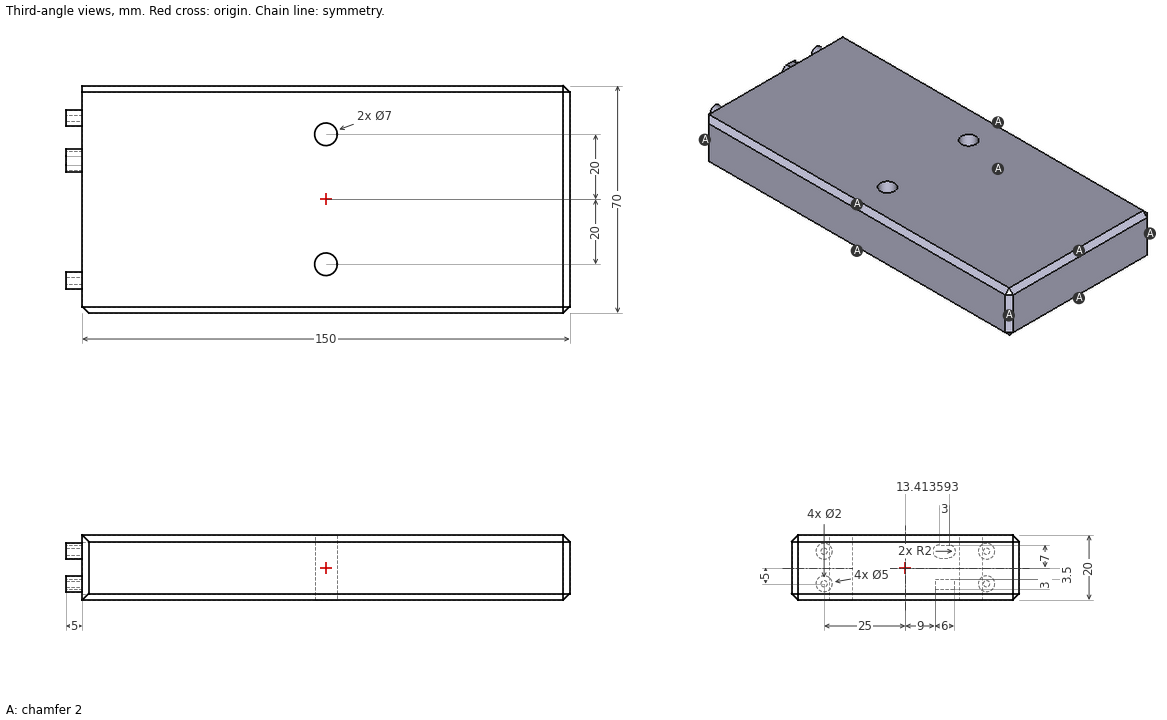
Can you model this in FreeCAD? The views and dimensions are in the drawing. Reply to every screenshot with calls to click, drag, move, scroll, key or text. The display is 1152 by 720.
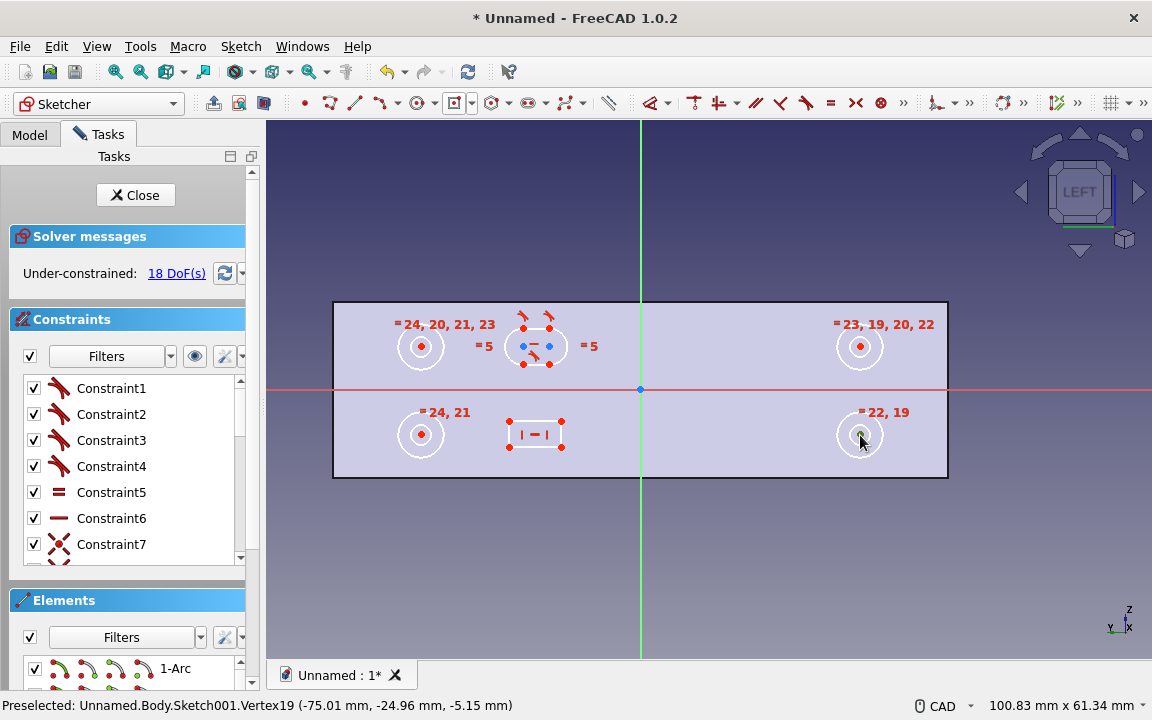
click(860, 347)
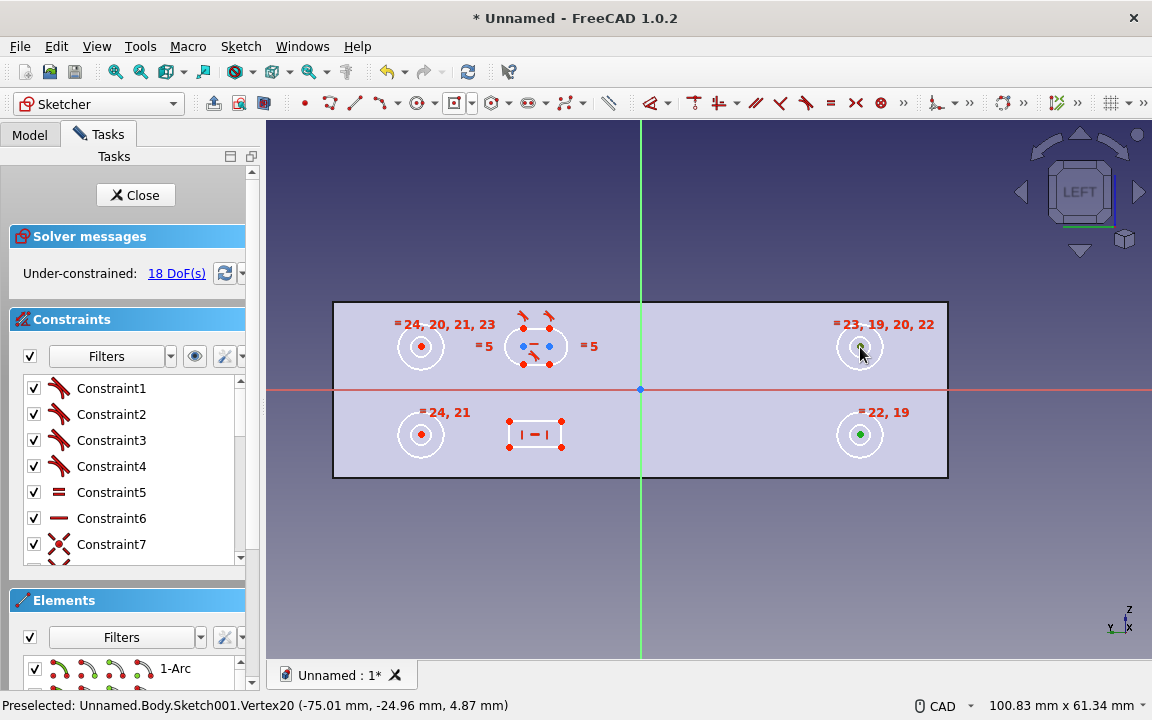
click(344, 390)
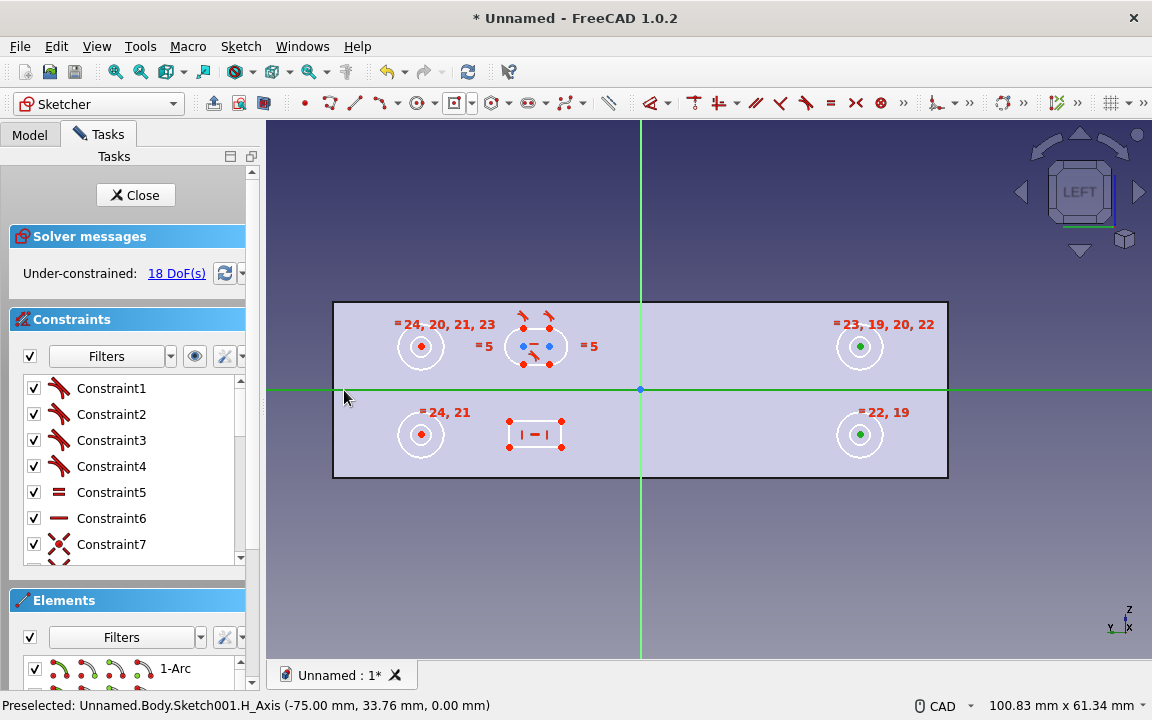
click(856, 104)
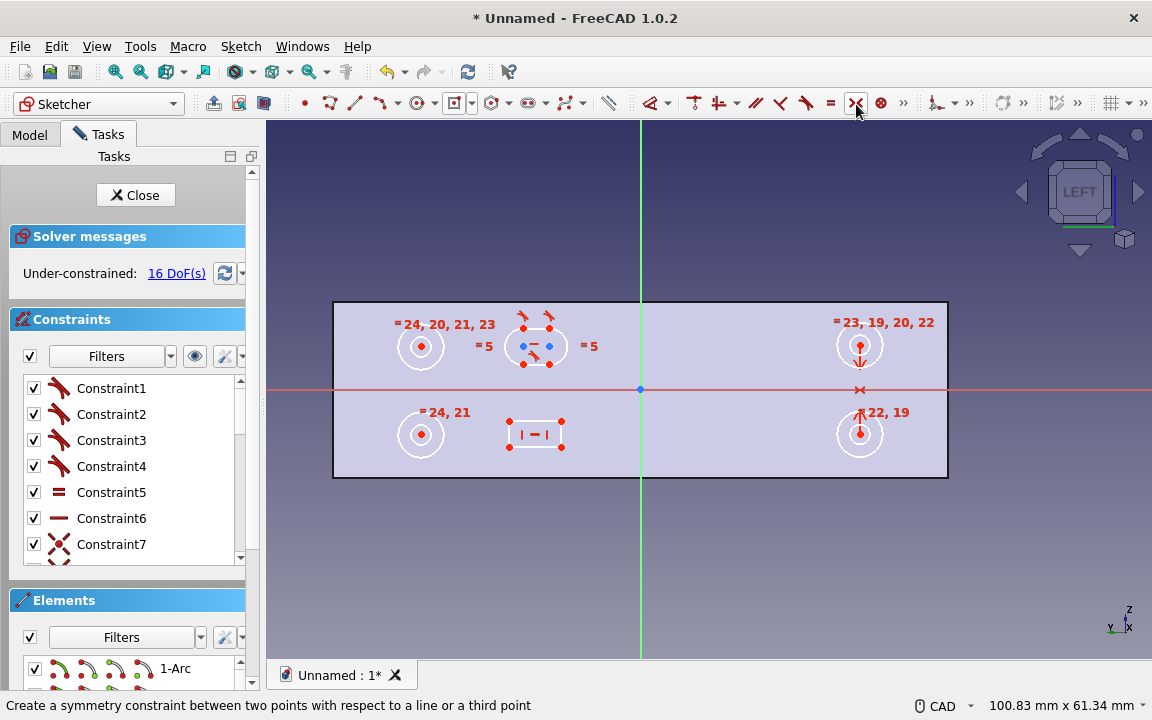
click(860, 345)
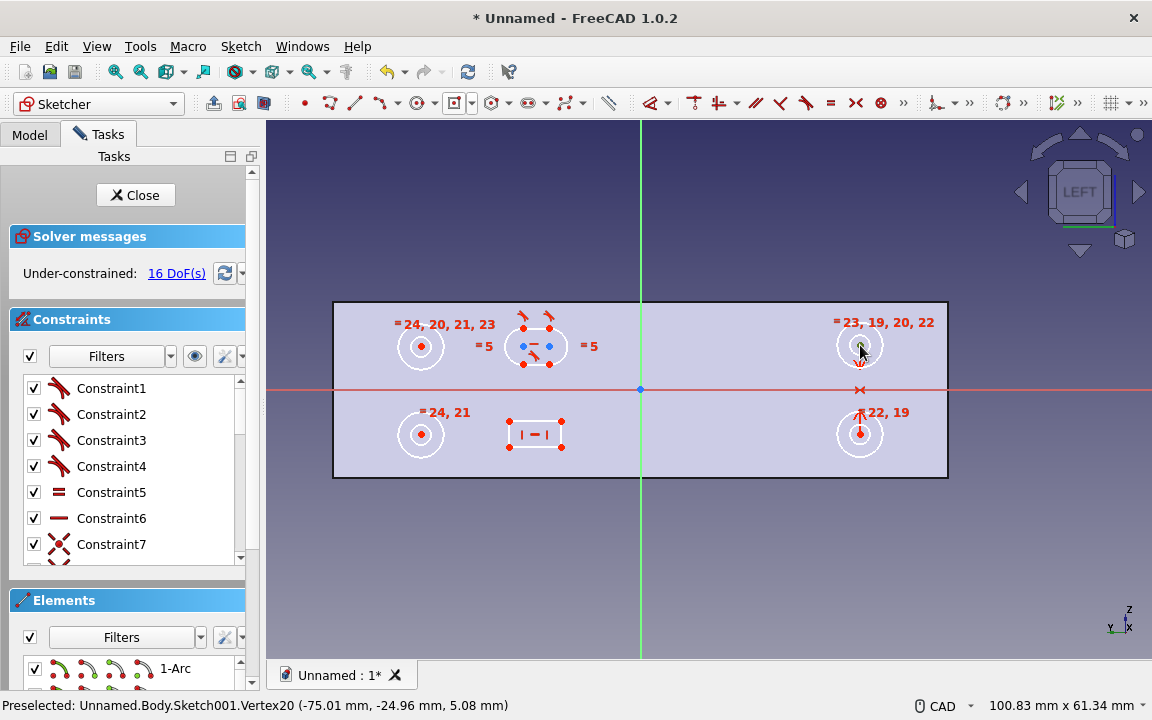
click(421, 347)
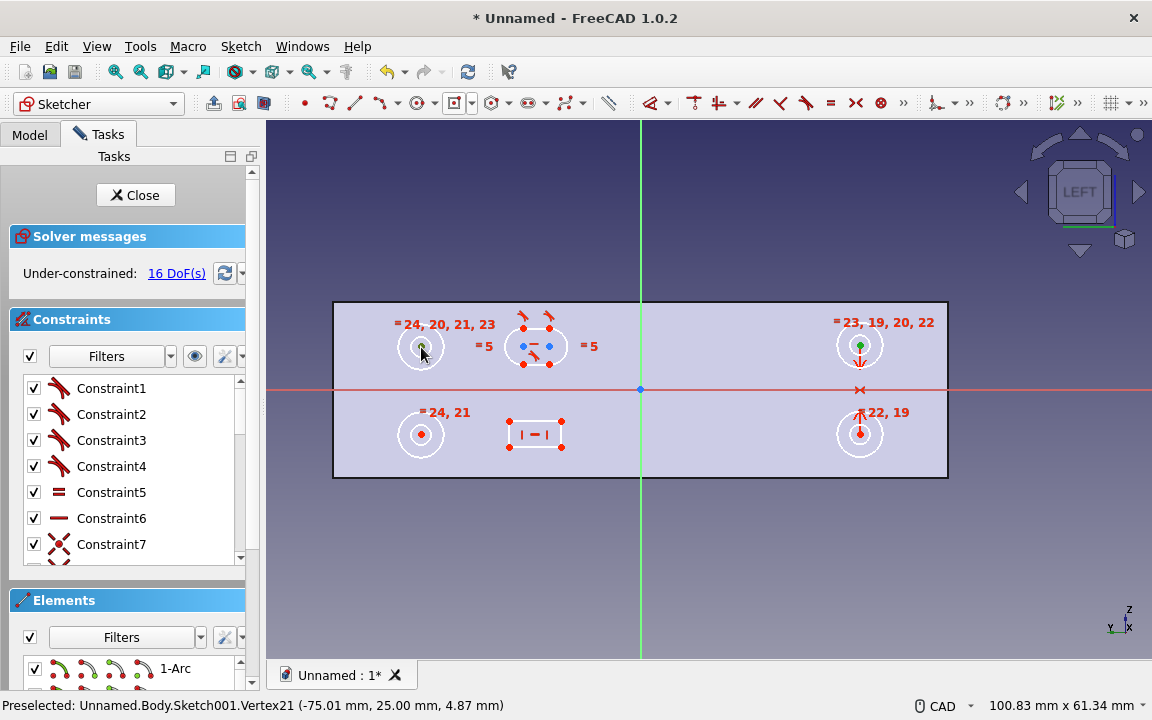
click(641, 596)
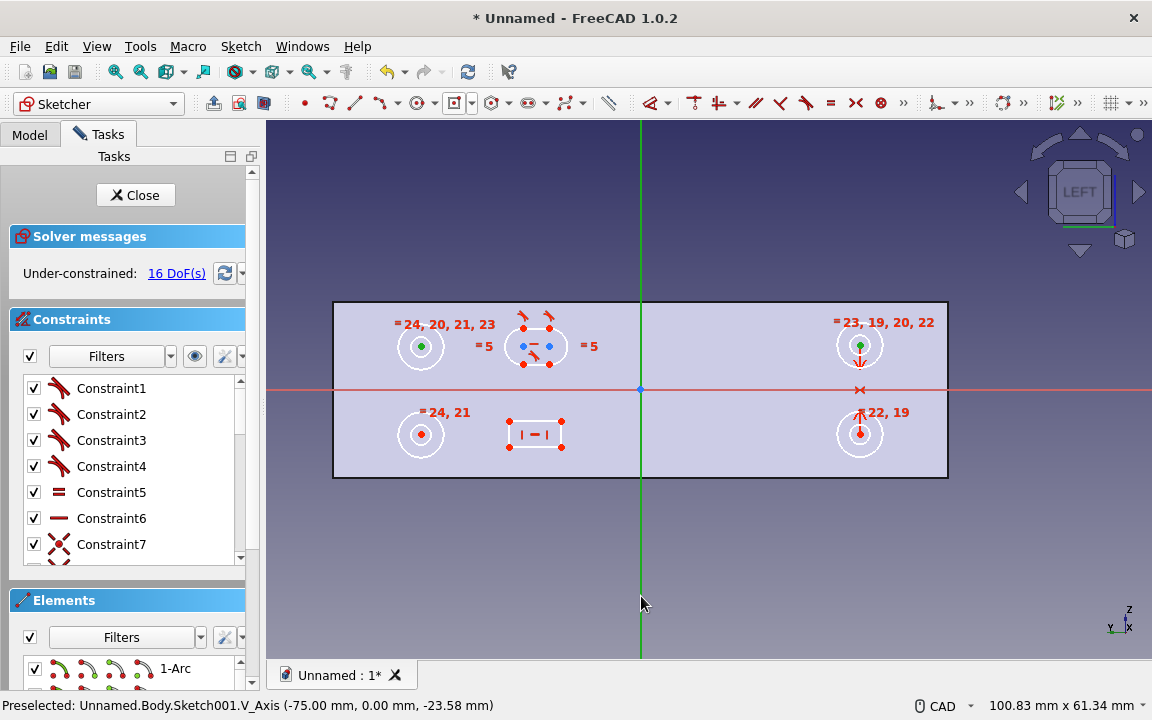
click(856, 104)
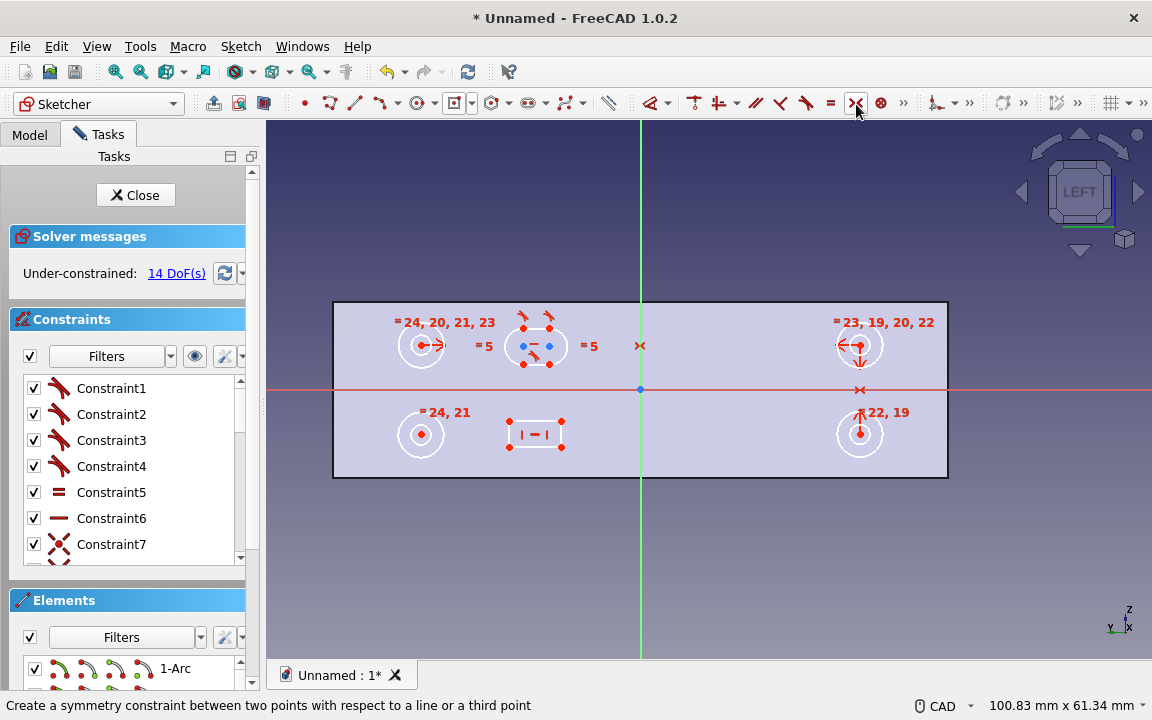
click(860, 434)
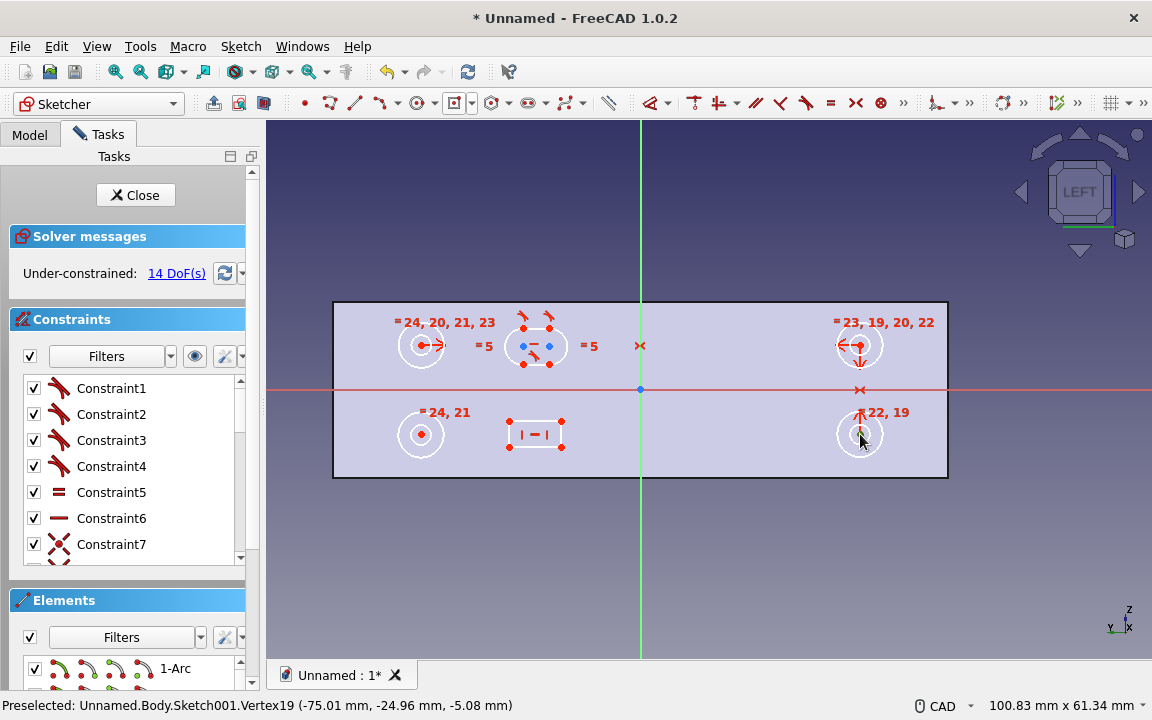
click(421, 435)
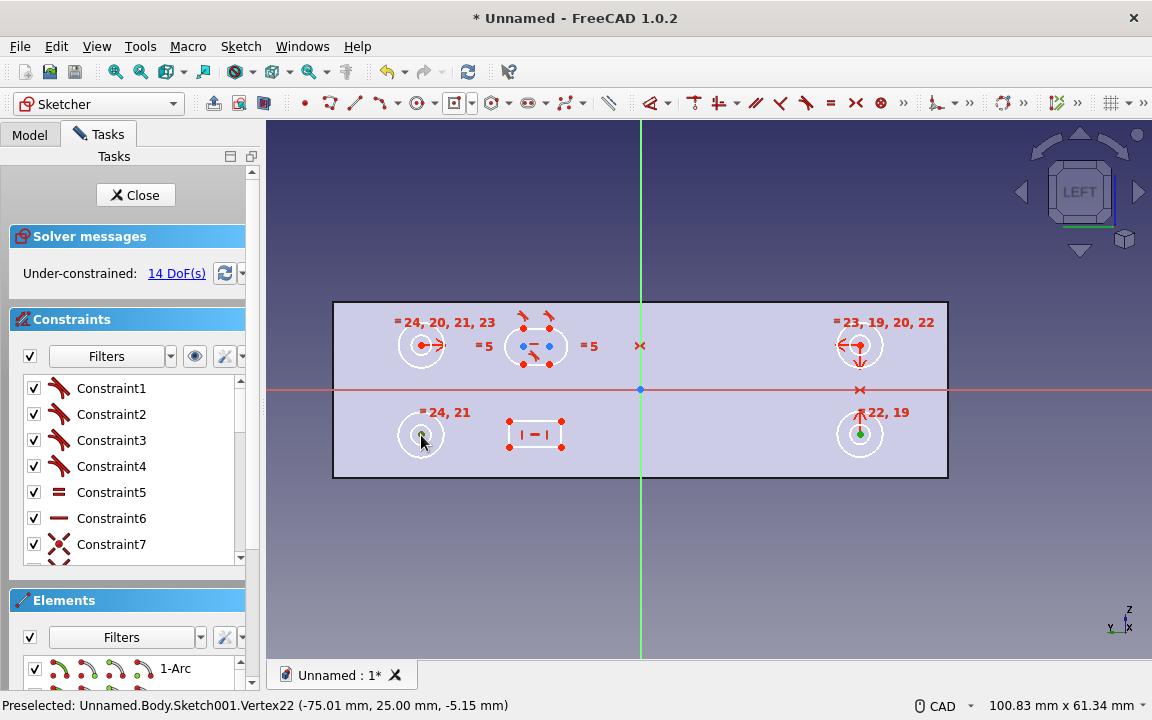
click(641, 596)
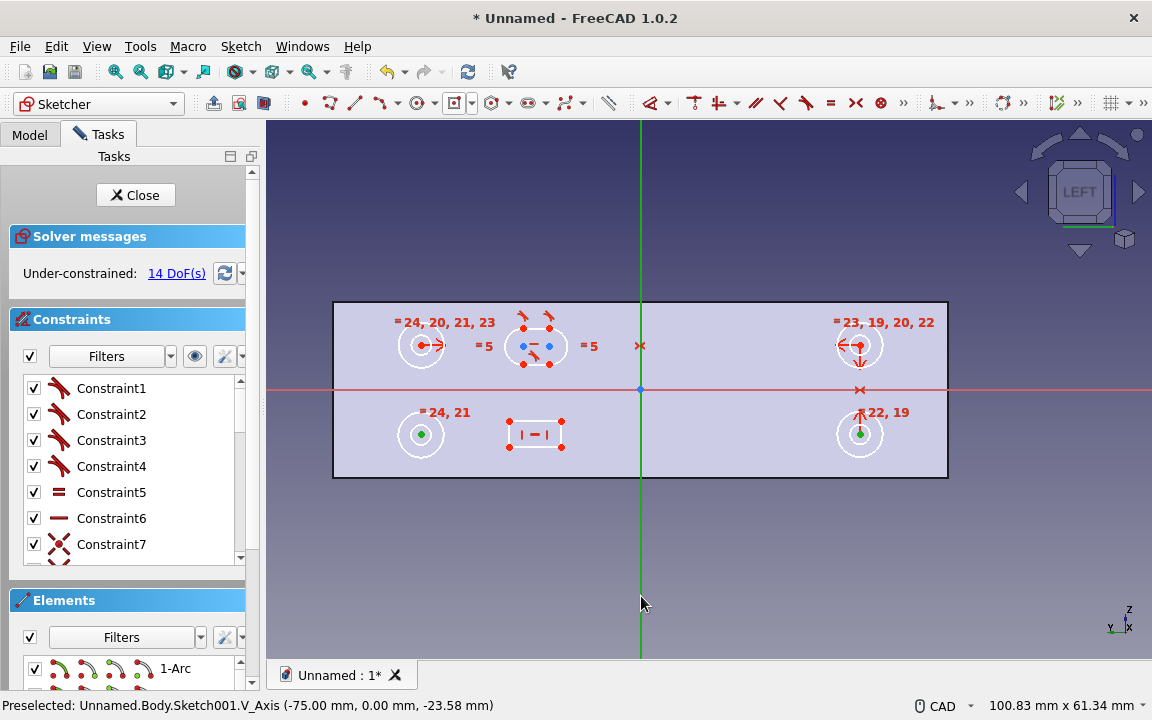
click(856, 104)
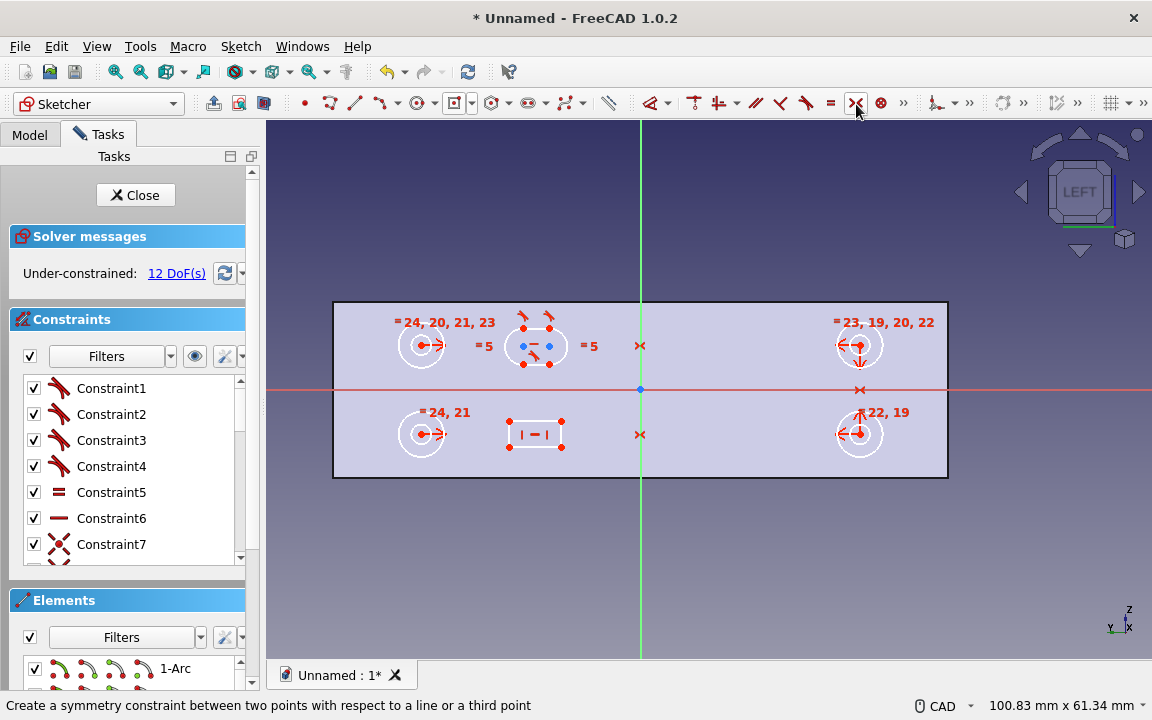
click(650, 104)